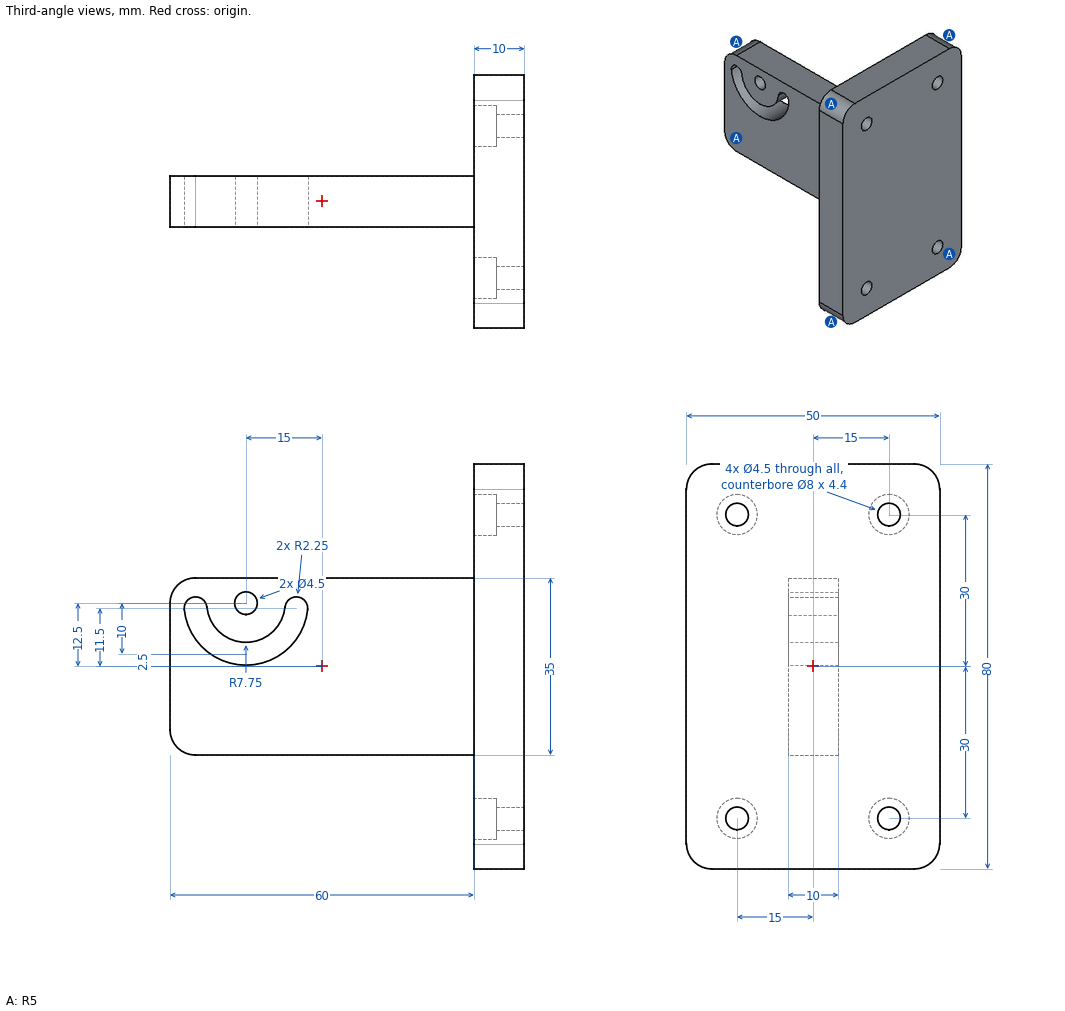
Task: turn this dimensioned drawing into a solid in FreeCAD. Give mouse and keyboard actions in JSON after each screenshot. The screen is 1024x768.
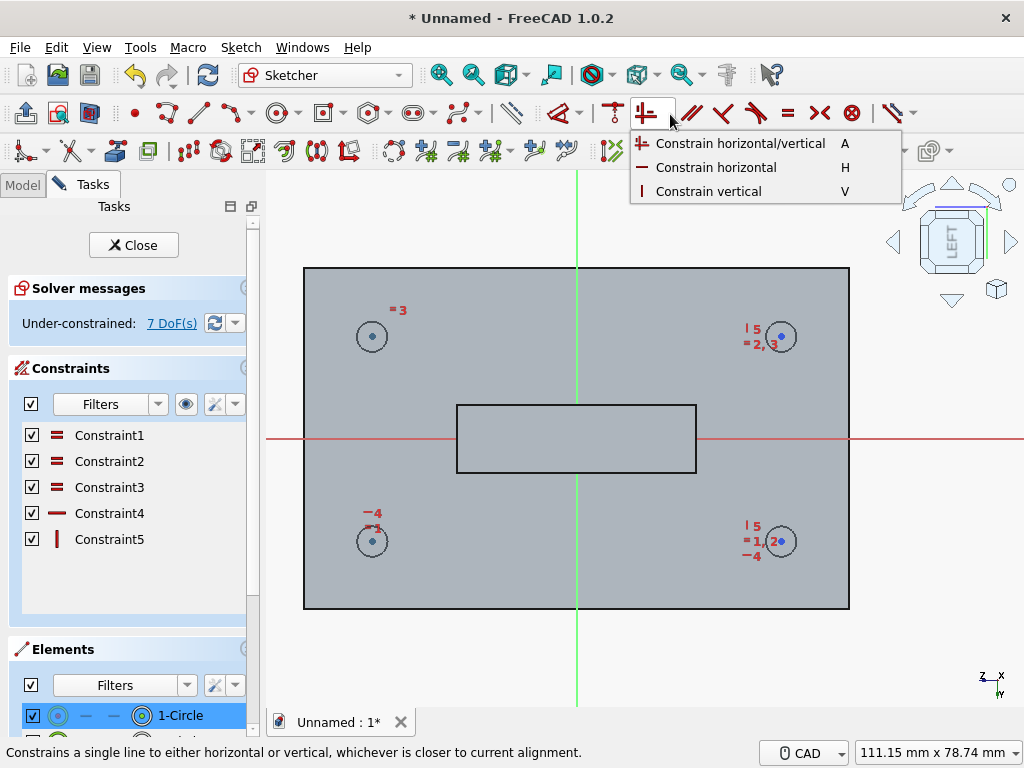
{"action": "left_click", "coordinate": [766, 191]}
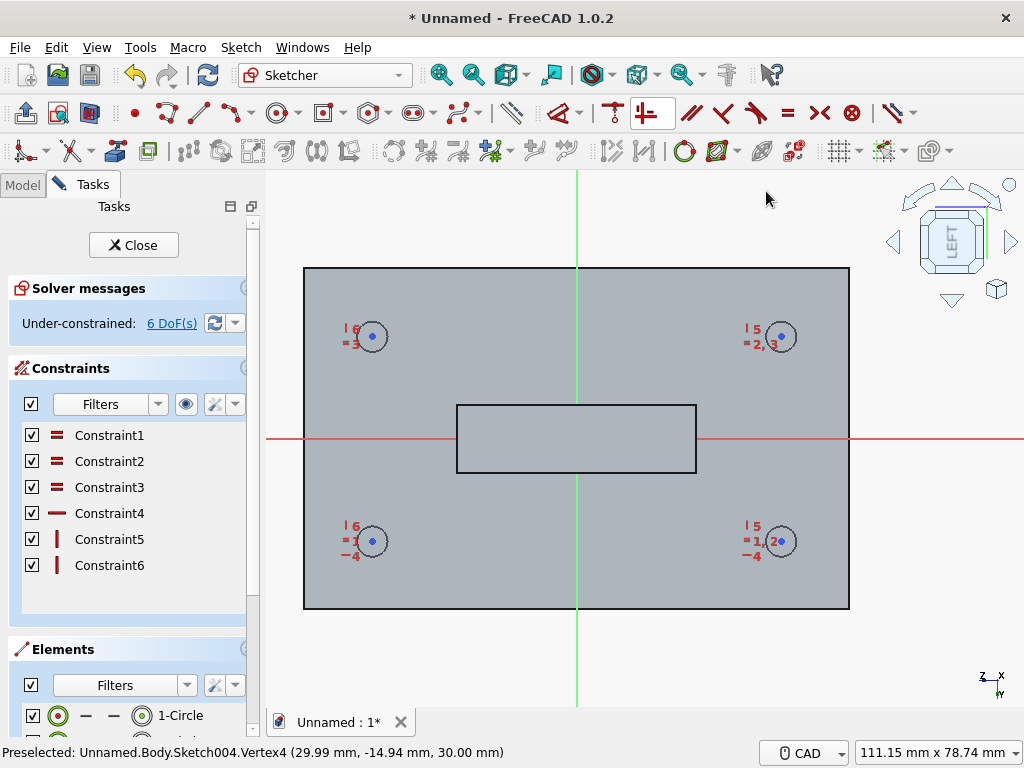
{"action": "left_click", "coordinate": [781, 337]}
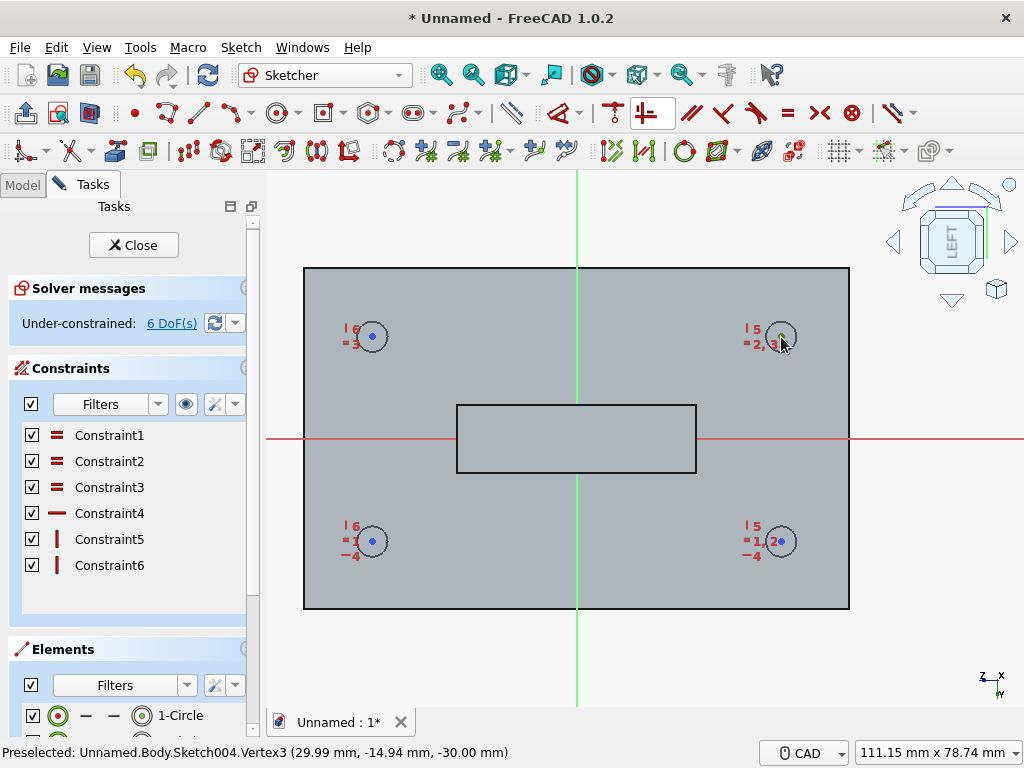
{"action": "left_click", "coordinate": [372, 337]}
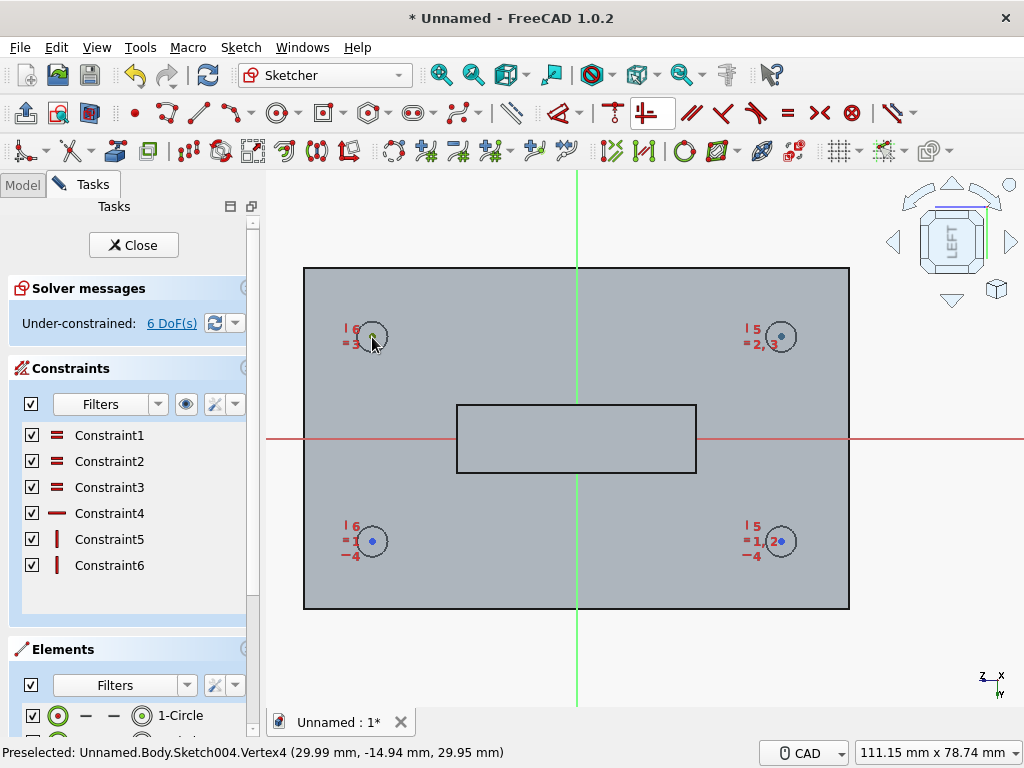
{"action": "left_click", "coordinate": [670, 114]}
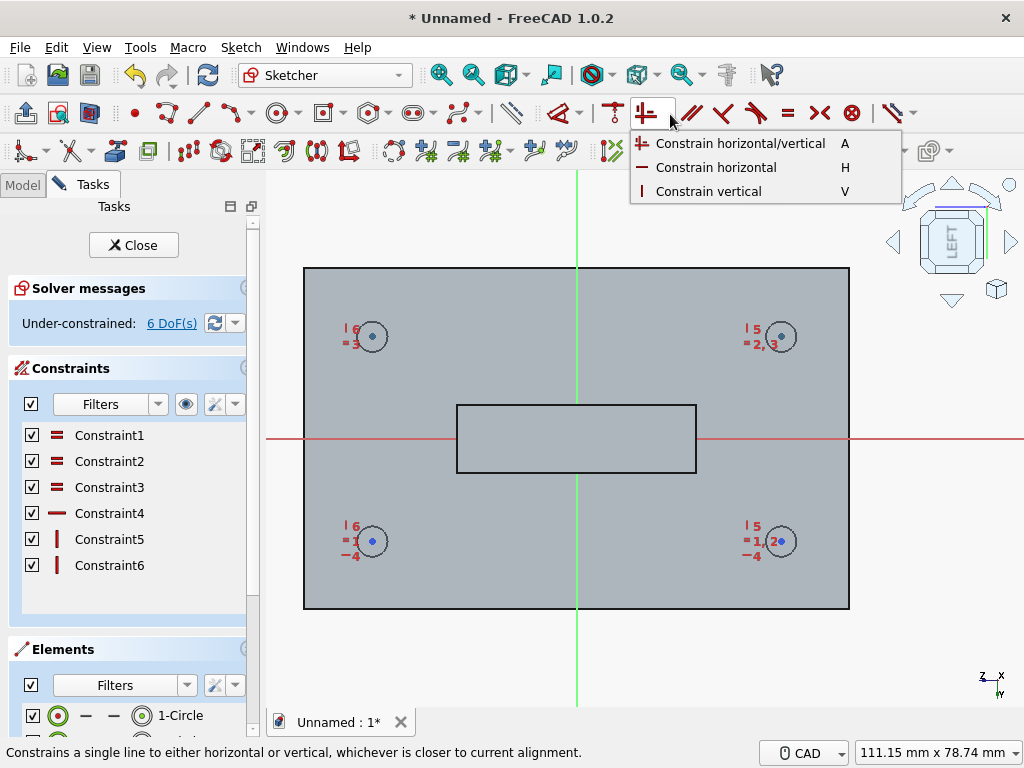
{"action": "left_click", "coordinate": [766, 167]}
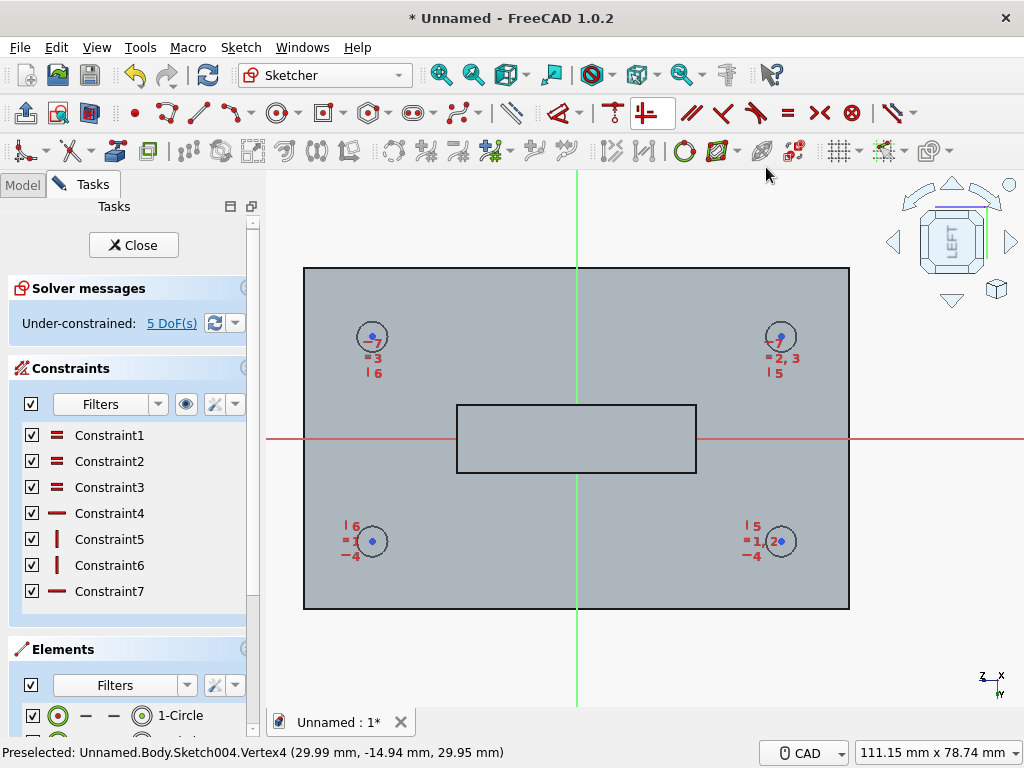
{"action": "left_click", "coordinate": [558, 114]}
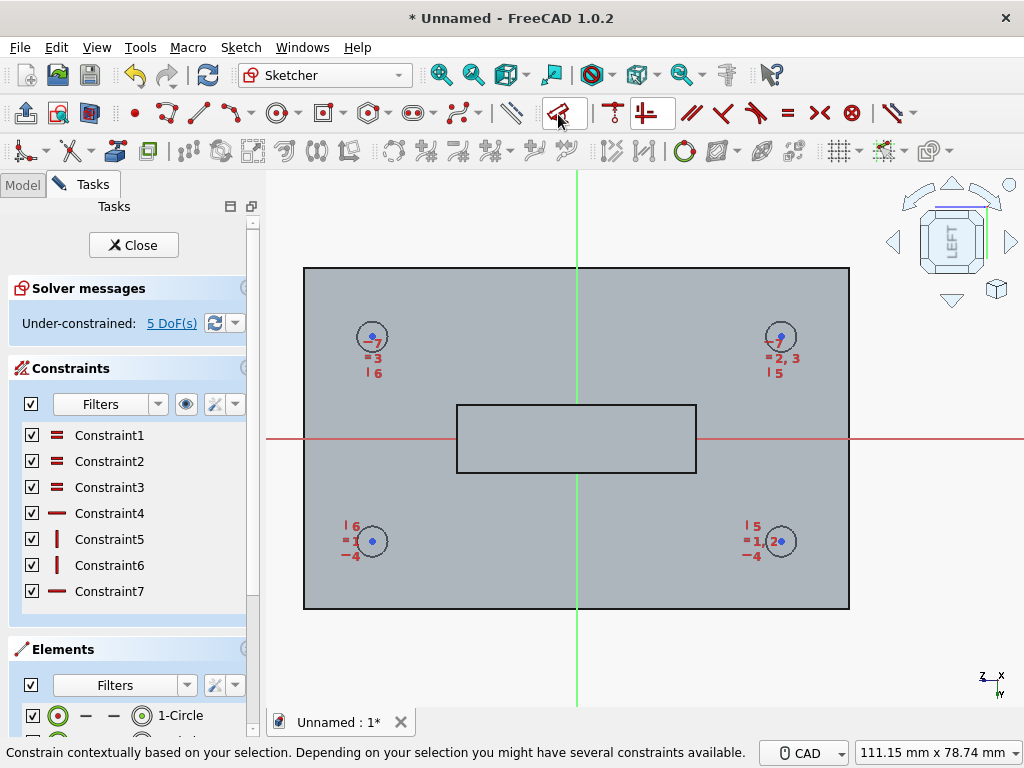
{"action": "scroll", "coordinate": [383, 531], "scroll_direction": "up", "scroll_amount": 2}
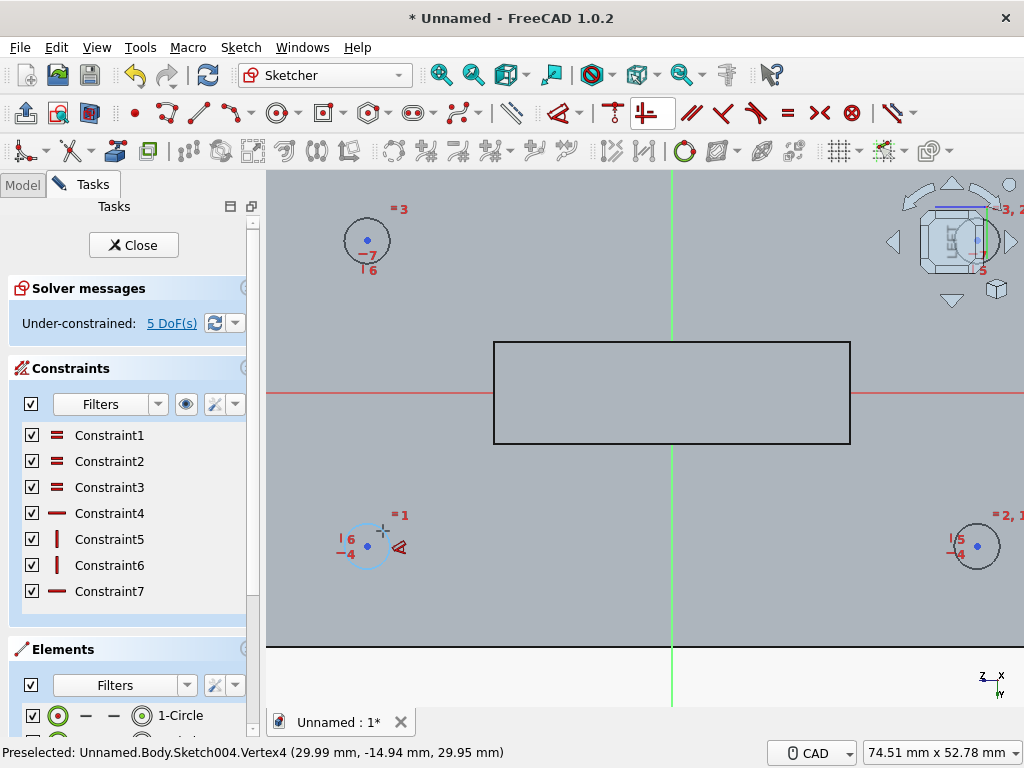
{"action": "left_click", "coordinate": [383, 530]}
{"action": "left_click", "coordinate": [405, 507]}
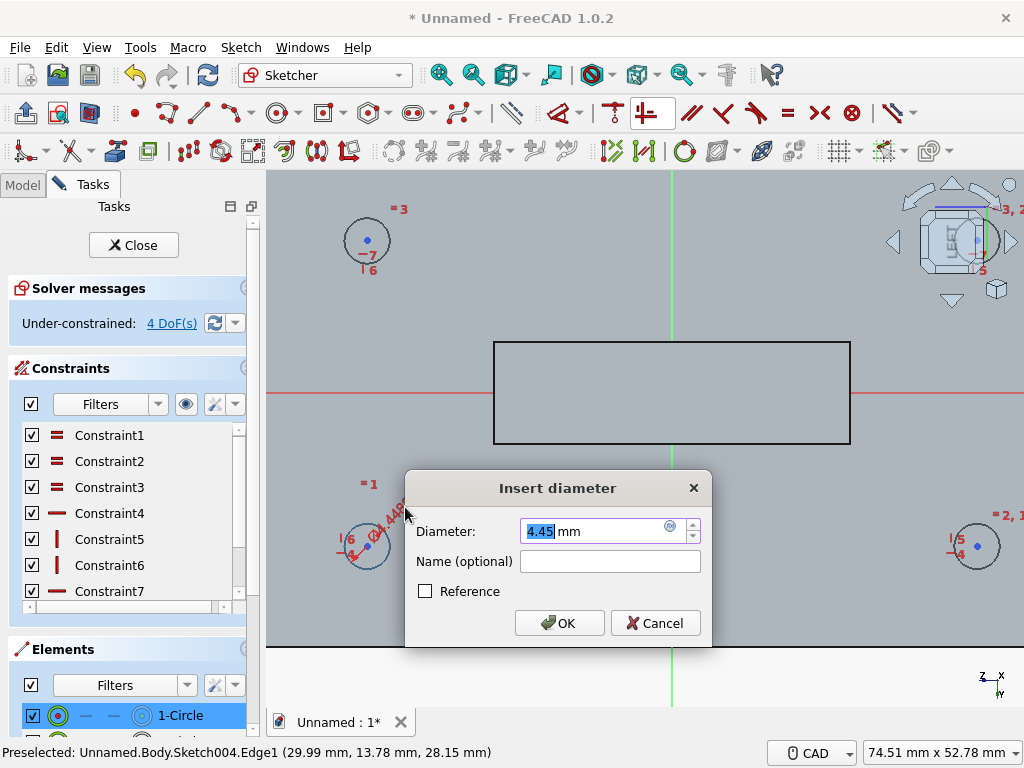
{"action": "type", "text": "4.5"}
{"action": "key", "text": "Return"}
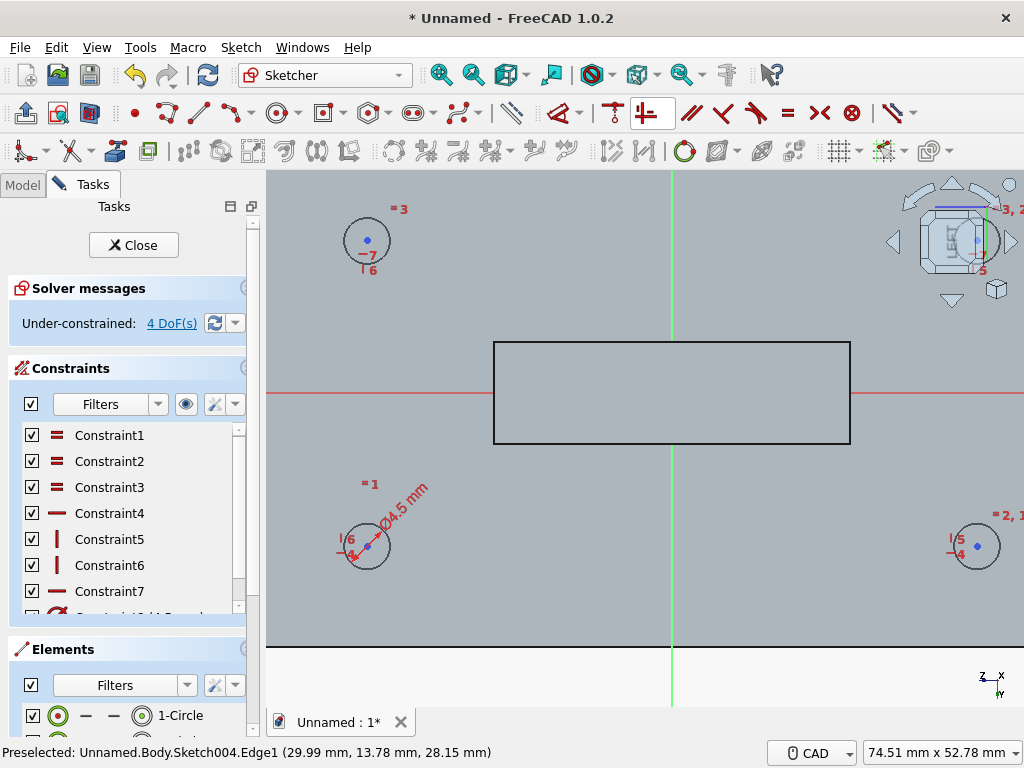
{"action": "left_click", "coordinate": [367, 546]}
{"action": "left_click", "coordinate": [519, 580]}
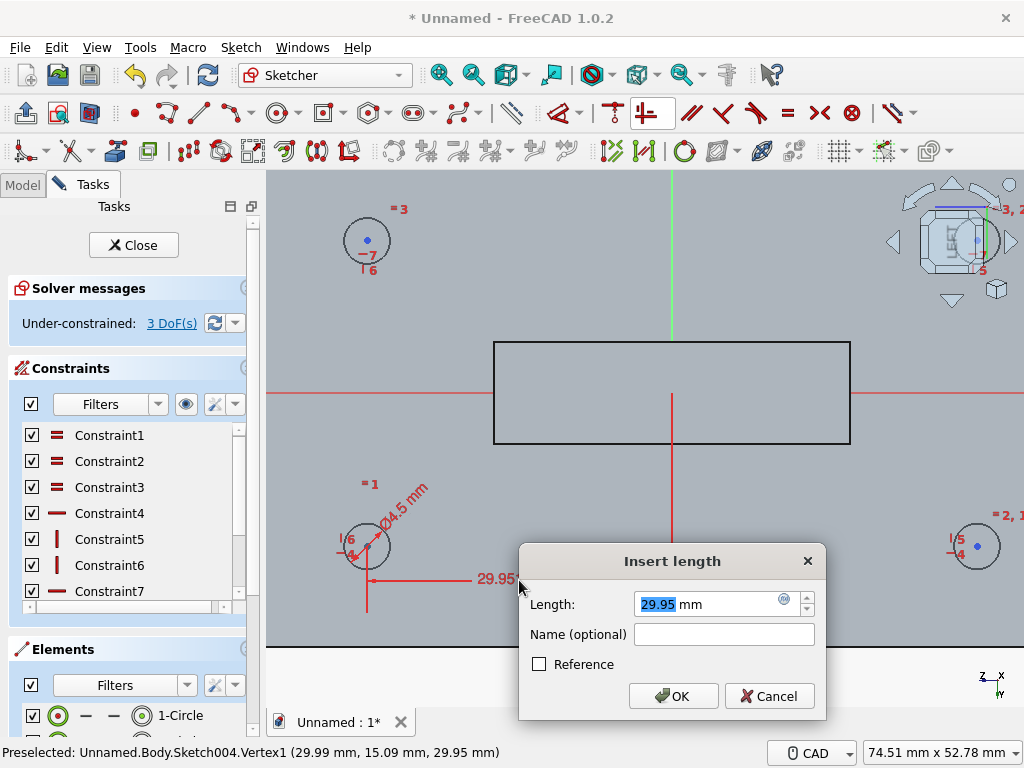
{"action": "type", "text": "30"}
{"action": "key", "text": "Return"}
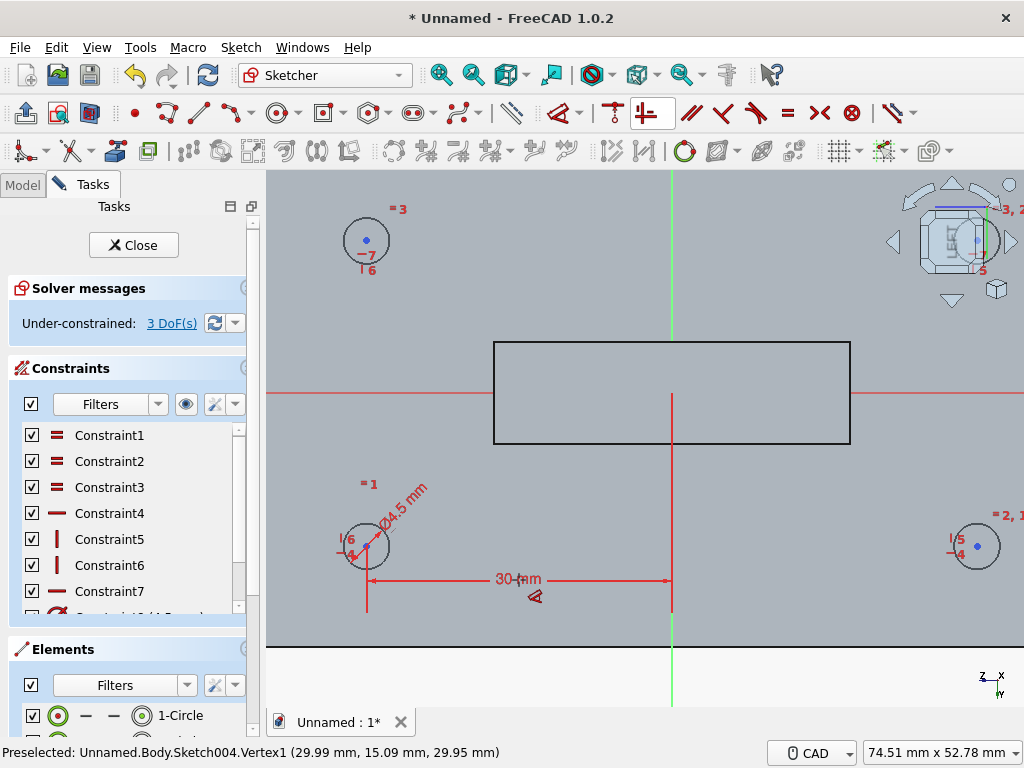
{"action": "left_click", "coordinate": [367, 546]}
{"action": "left_click", "coordinate": [333, 470]}